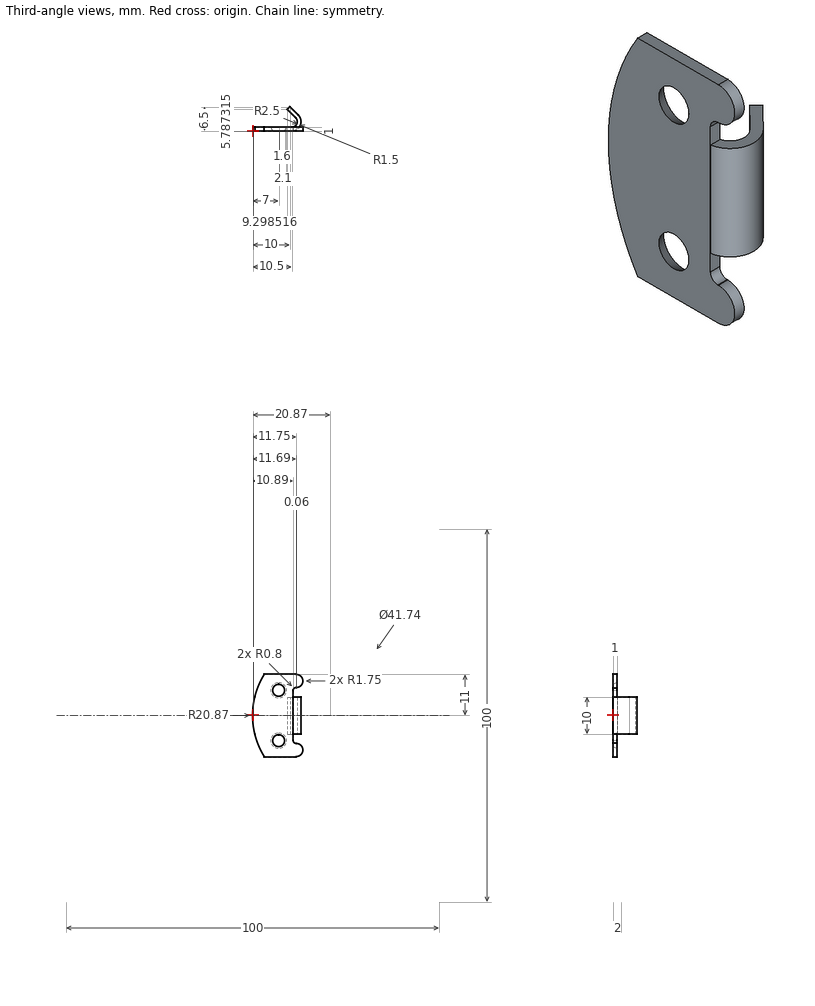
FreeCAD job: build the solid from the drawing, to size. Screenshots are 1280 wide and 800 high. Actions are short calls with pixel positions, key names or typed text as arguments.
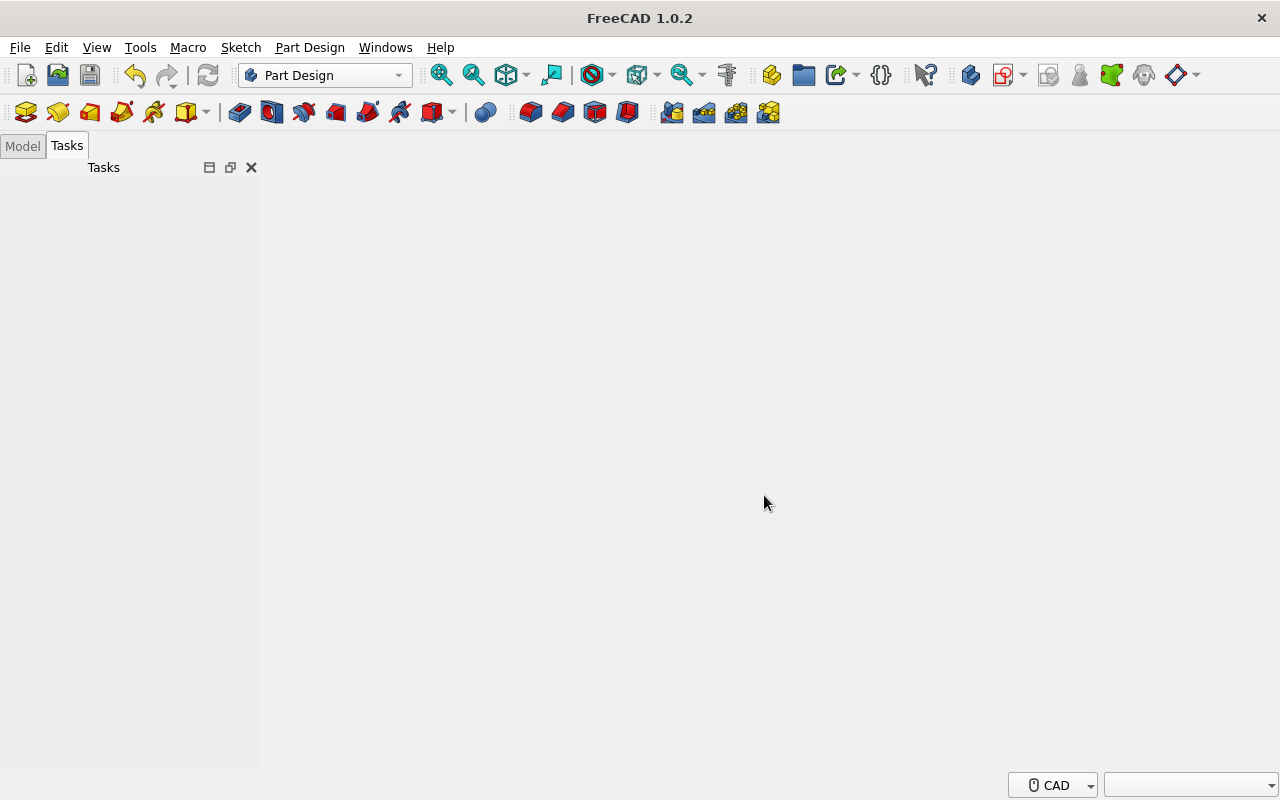
key(ctrl+n)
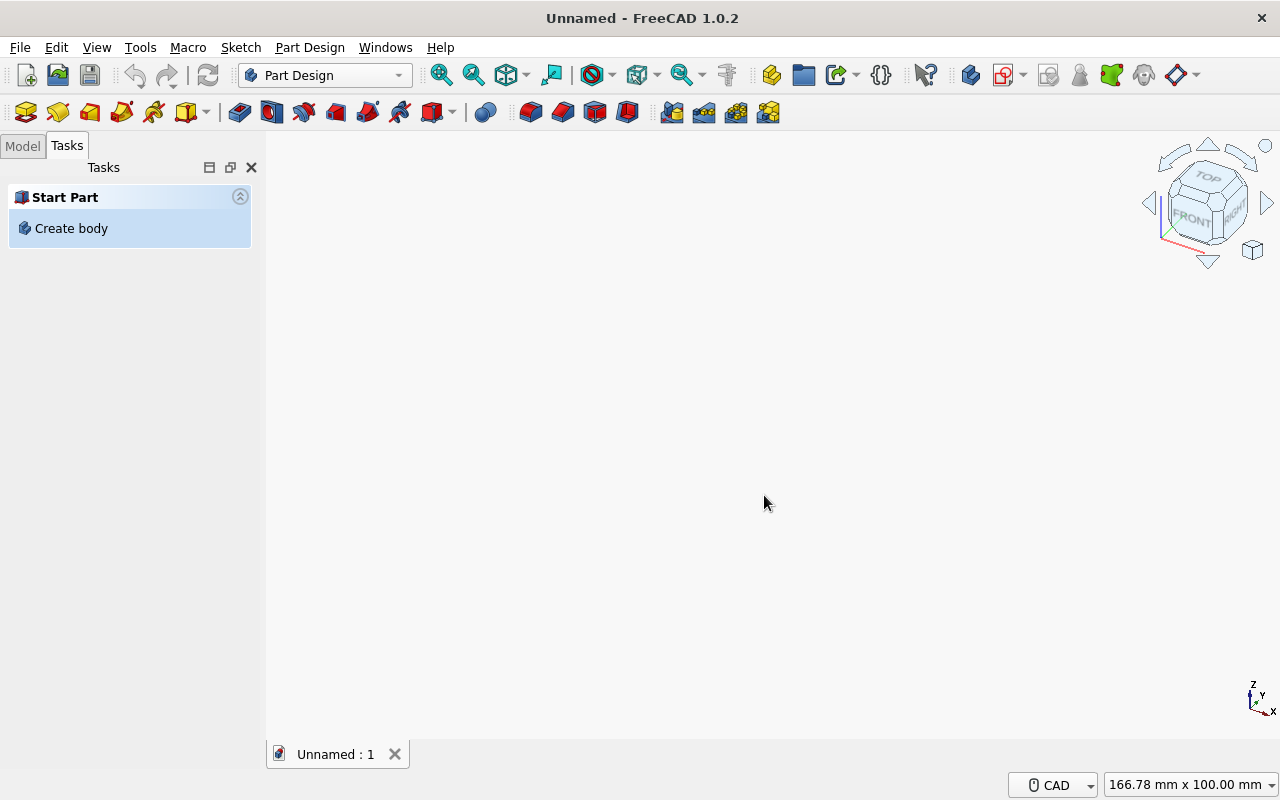
click(1004, 76)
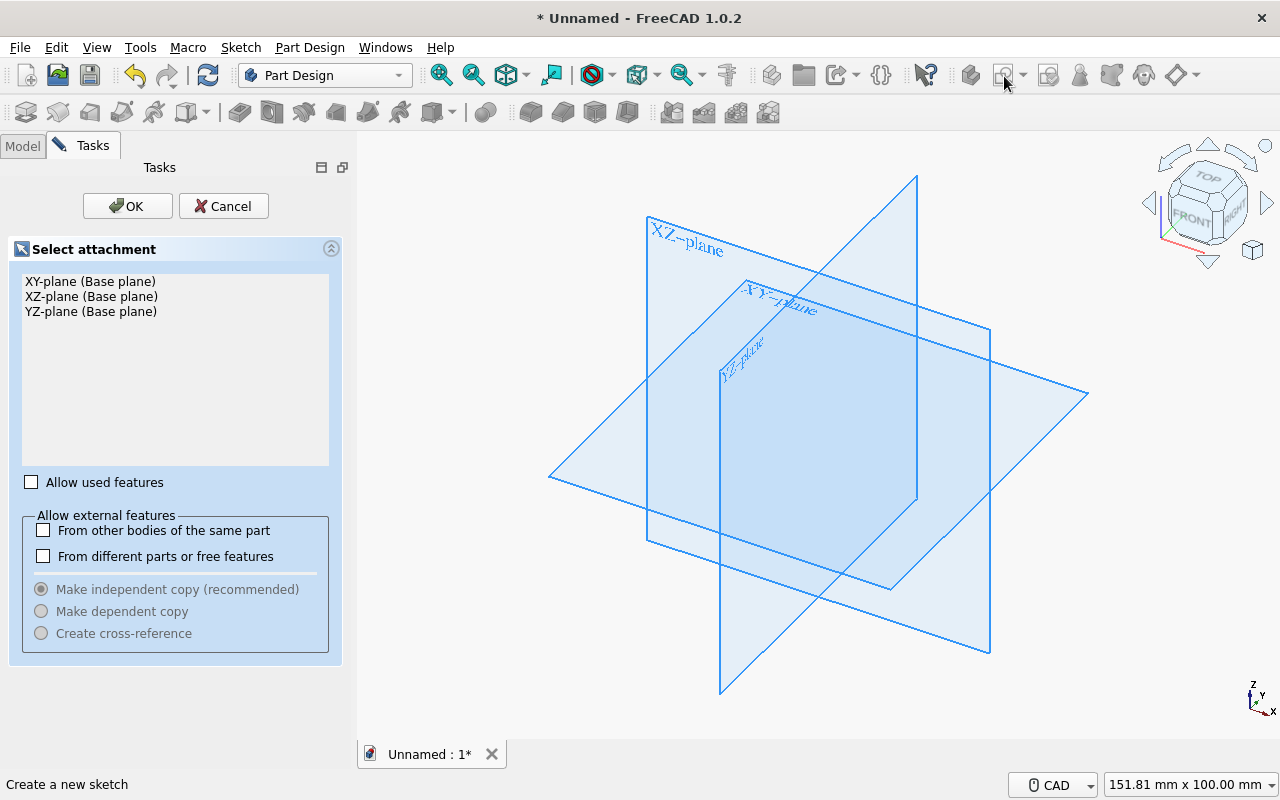
click(82, 282)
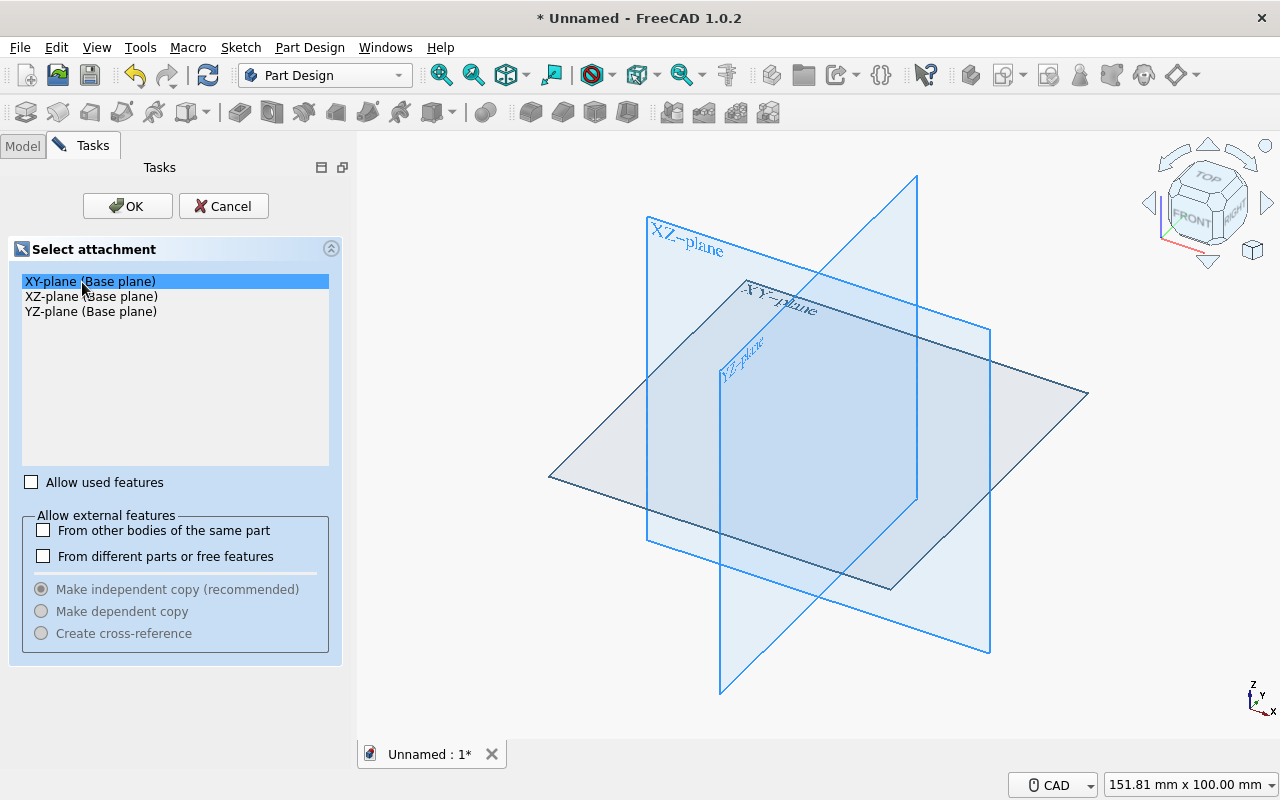
click(128, 206)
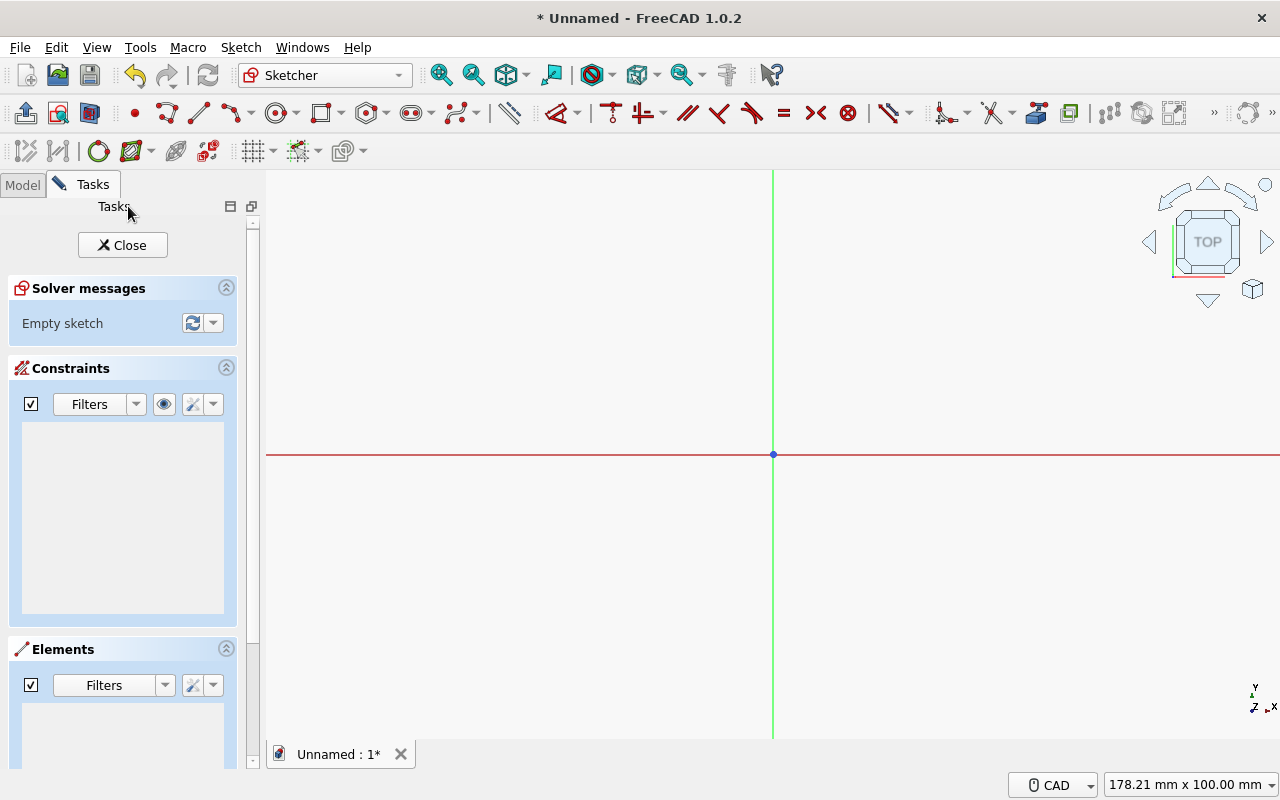
scroll(826, 433, up, 10)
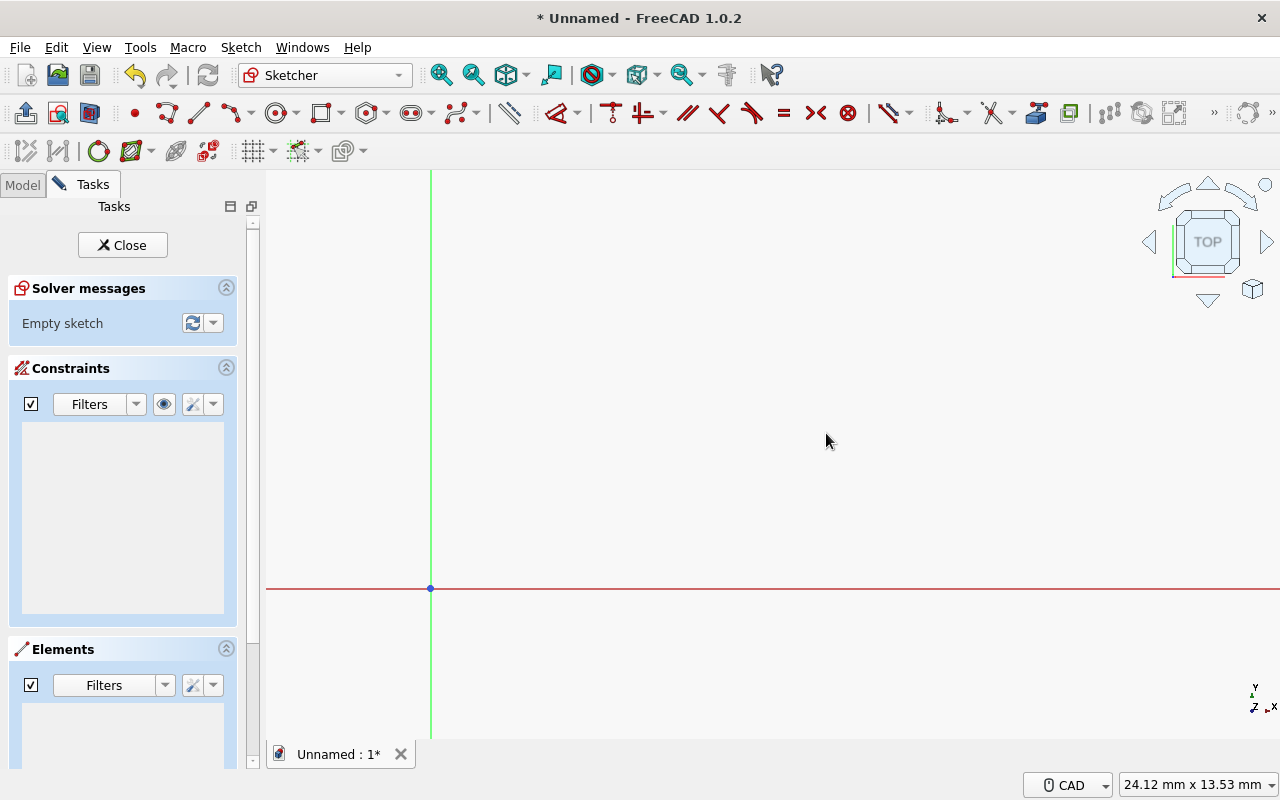
click(168, 114)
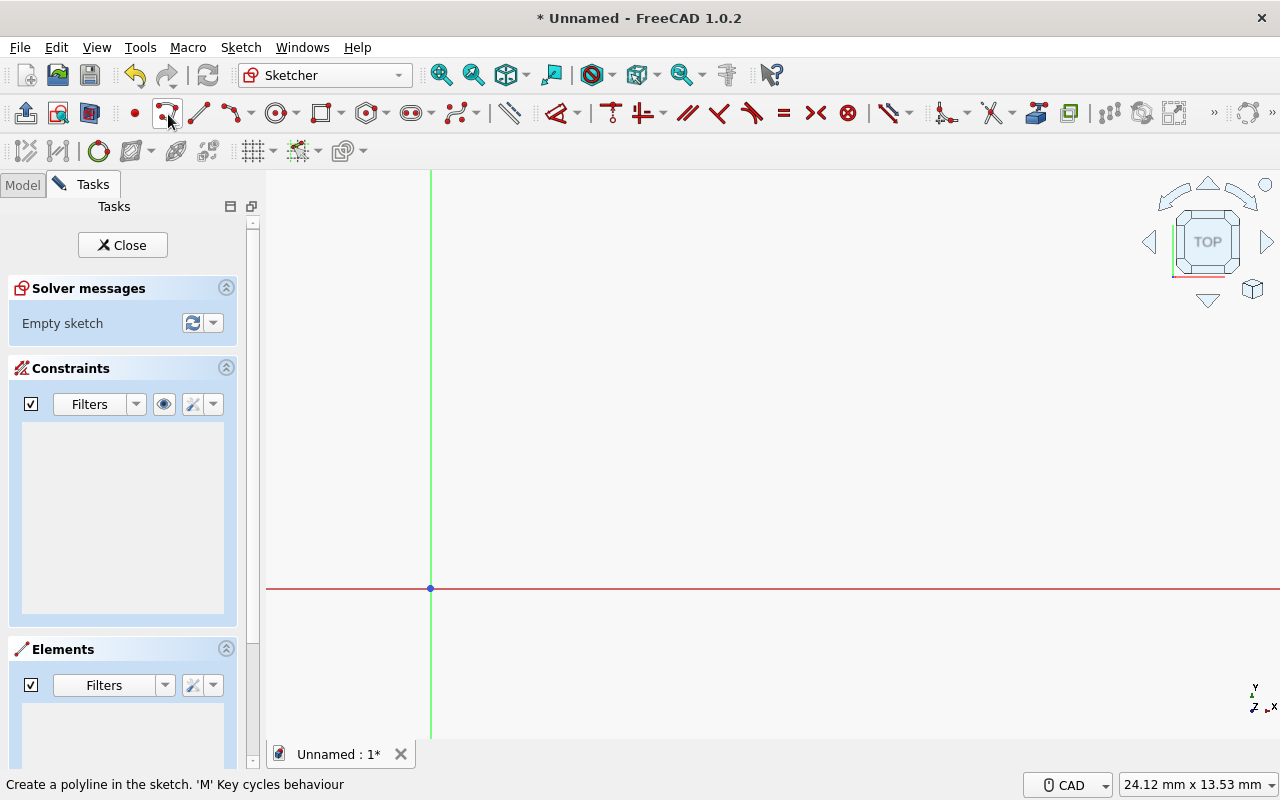
click(946, 409)
click(851, 316)
click(822, 346)
click(917, 439)
right_click(917, 439)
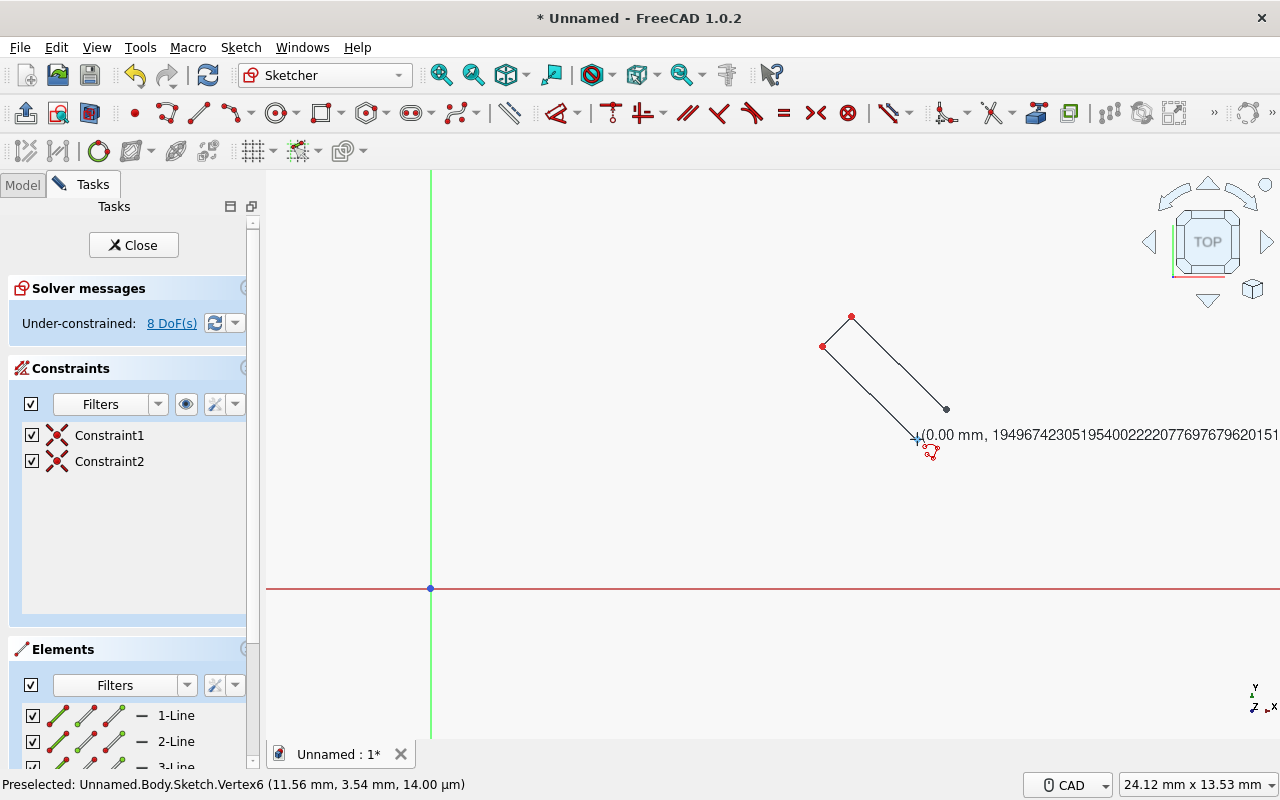
click(872, 547)
click(431, 547)
click(431, 589)
click(872, 580)
right_click(872, 580)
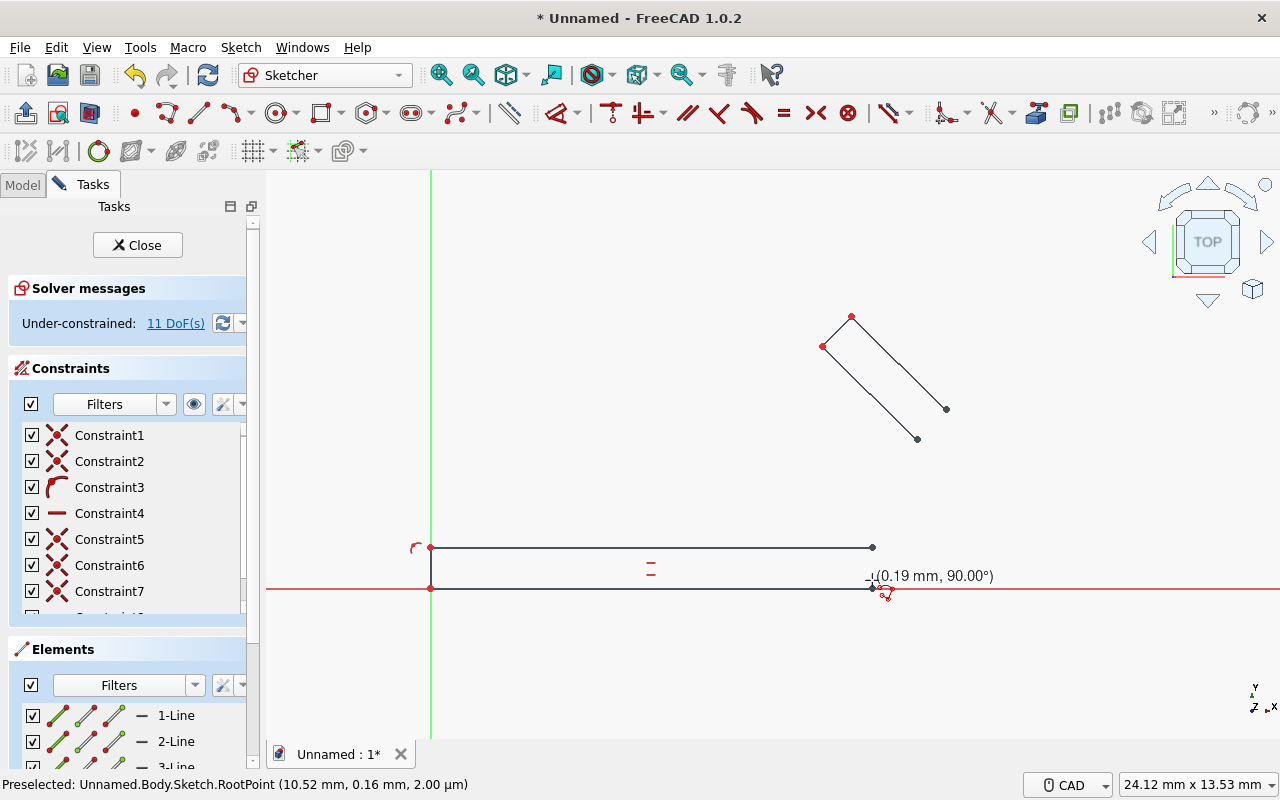
click(232, 114)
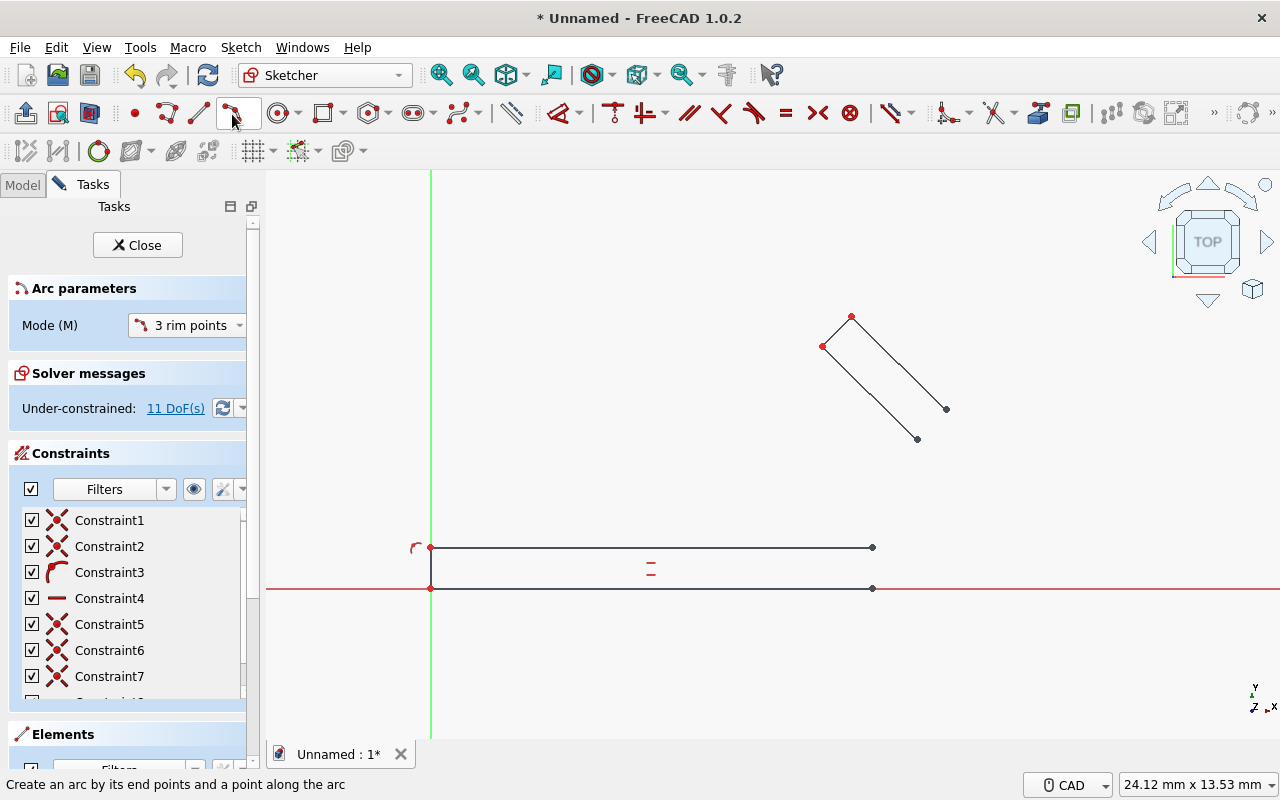
click(917, 440)
click(872, 548)
click(931, 508)